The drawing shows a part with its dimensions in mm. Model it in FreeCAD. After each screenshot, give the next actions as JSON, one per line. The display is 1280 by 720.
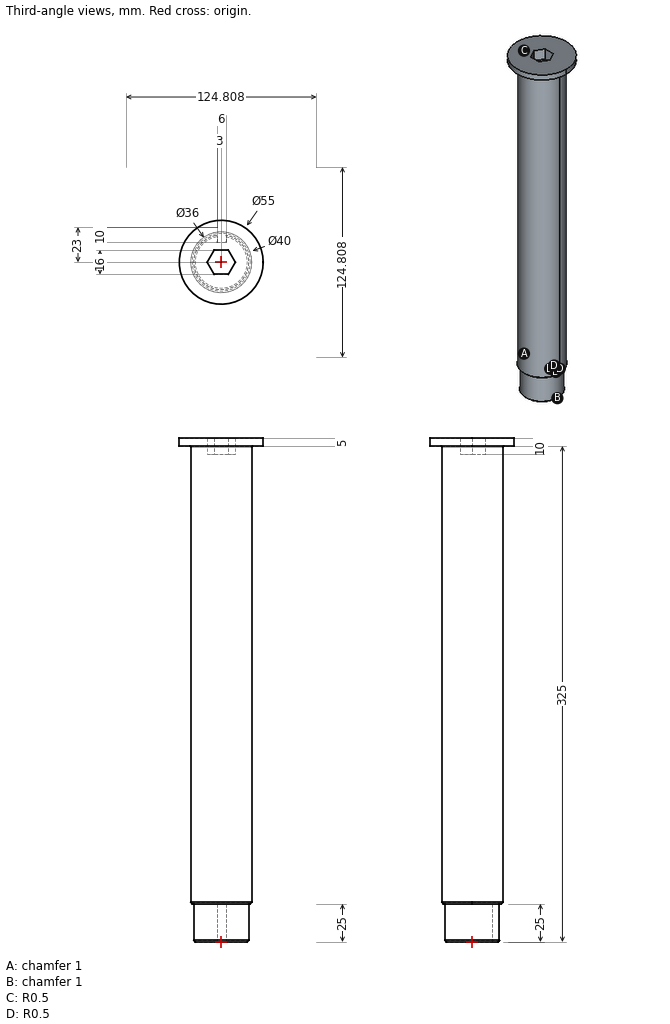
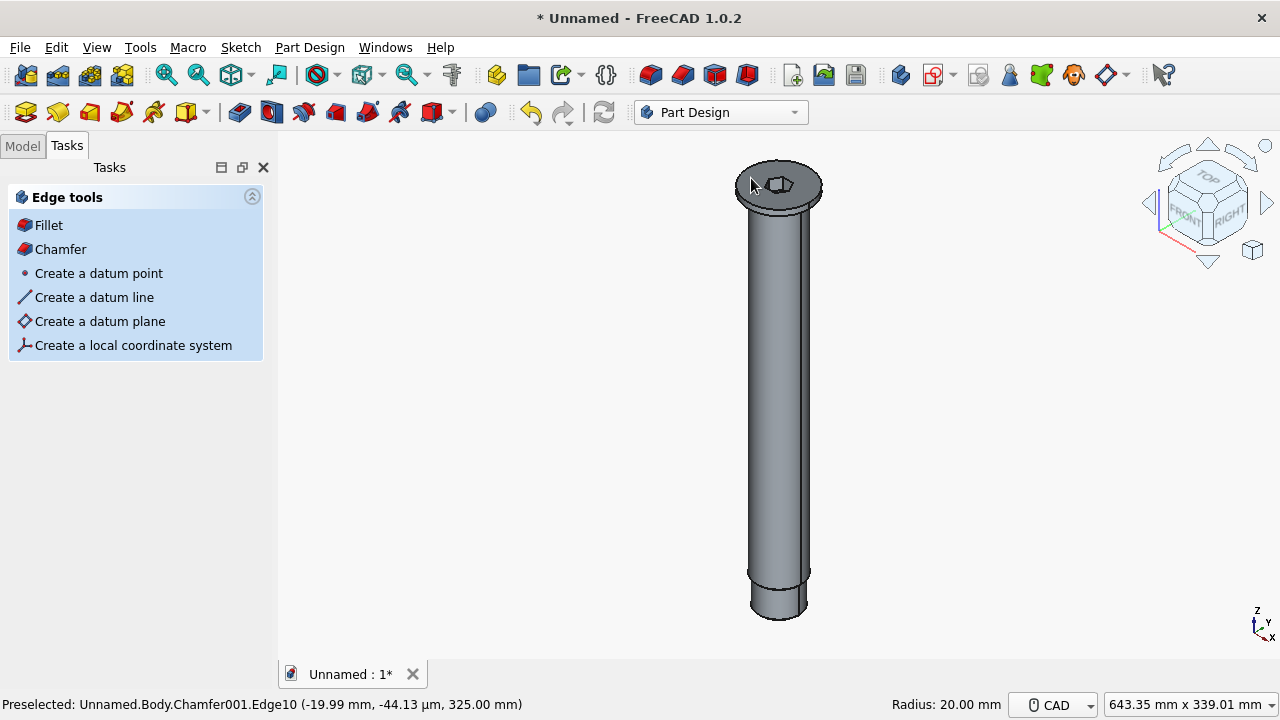
{"action": "left_click", "coordinate": [652, 76]}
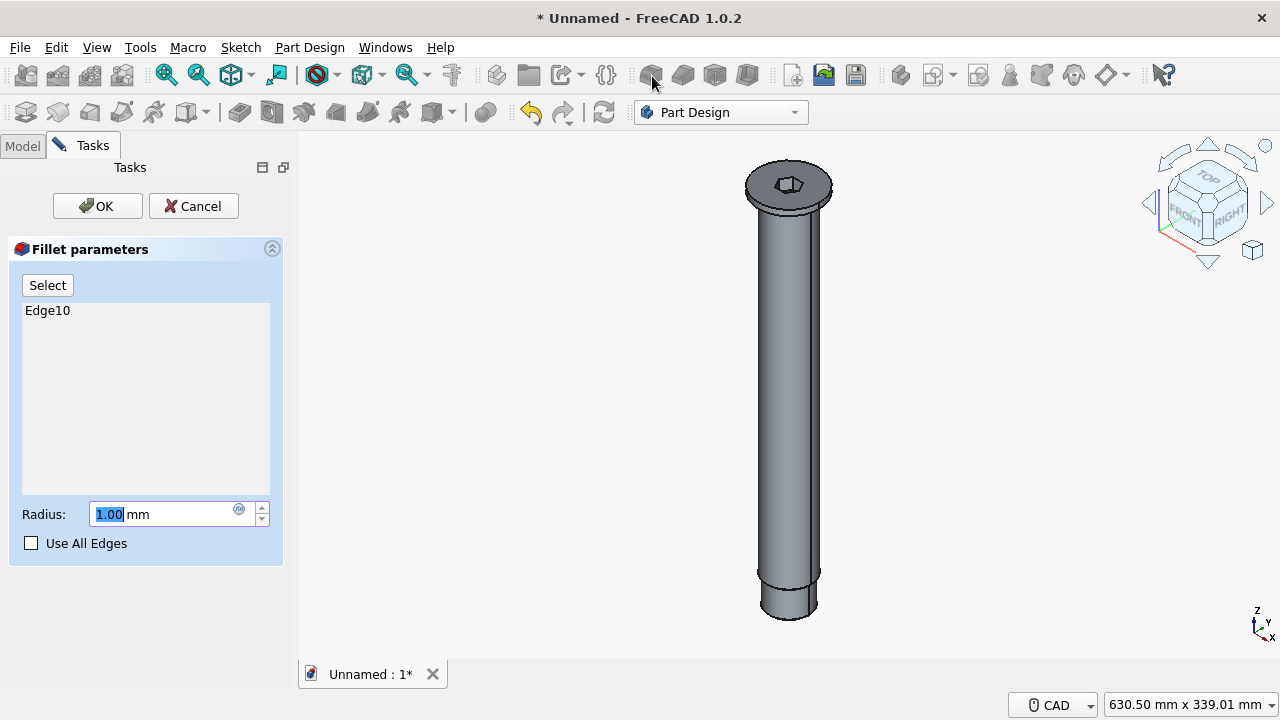
{"action": "type", "text": "0.5"}
{"action": "key", "text": "Tab"}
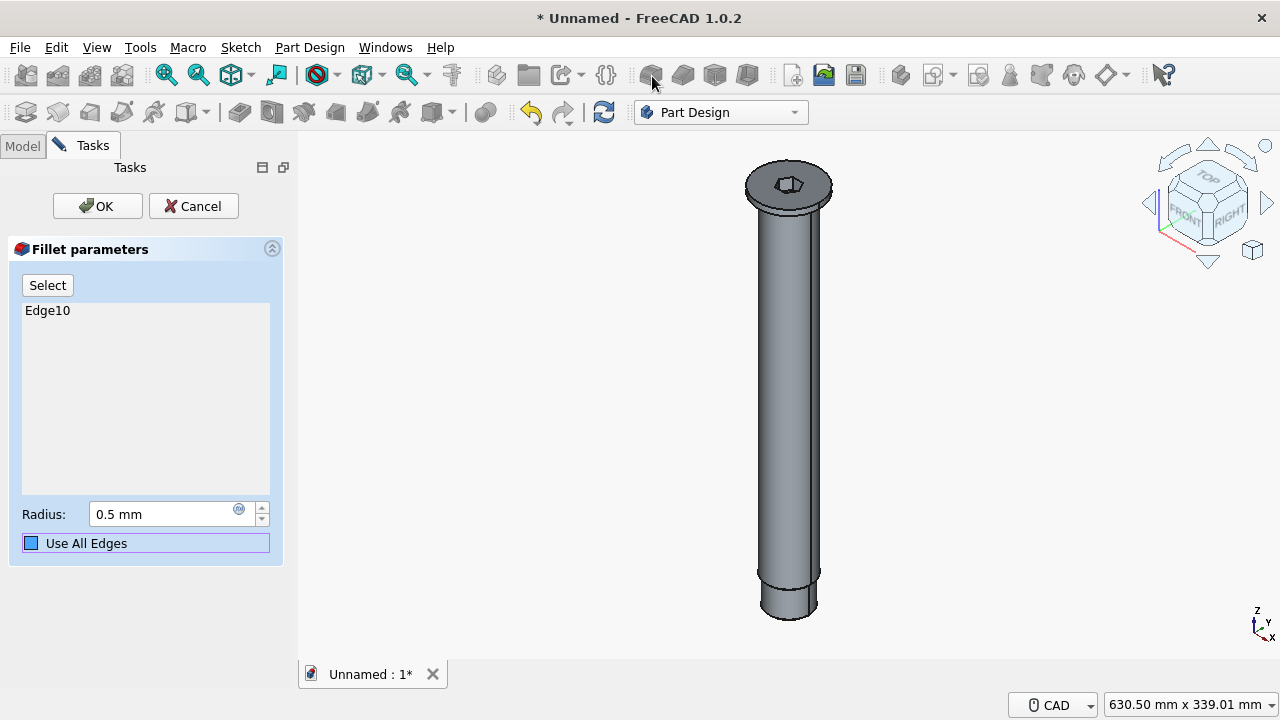
{"action": "left_click", "coordinate": [98, 206]}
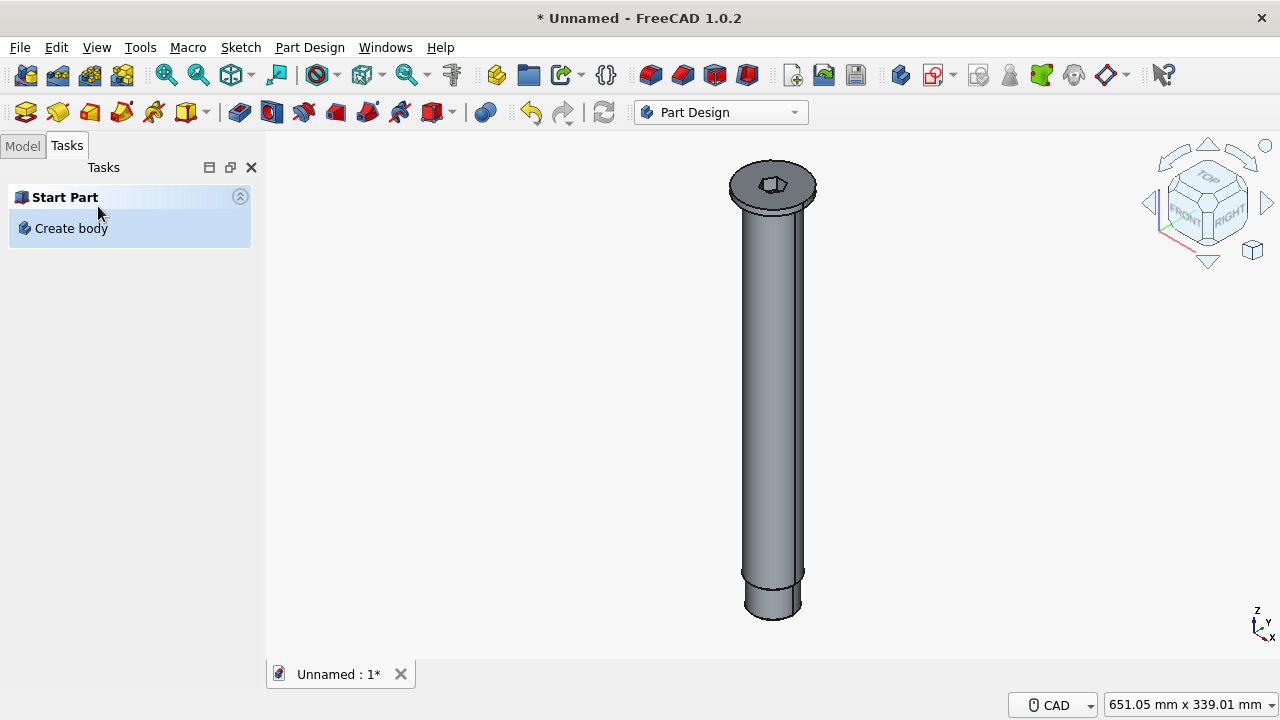
{"action": "left_click", "coordinate": [934, 76]}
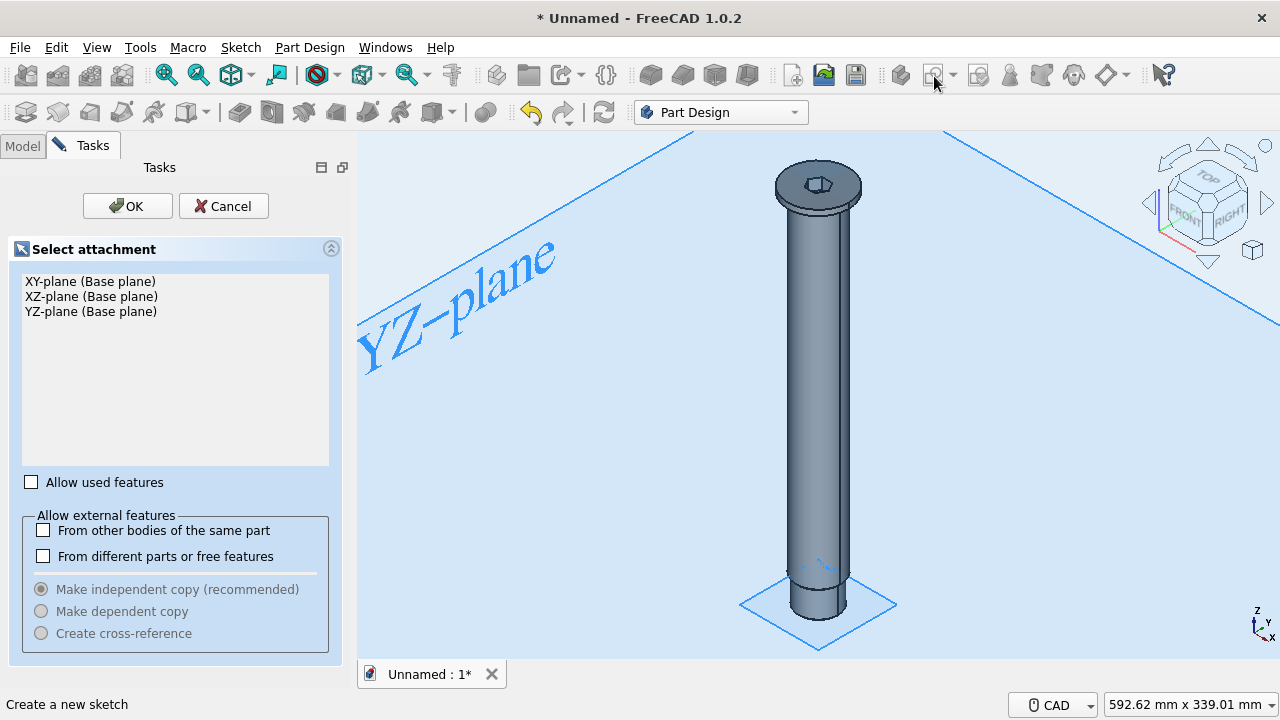
{"action": "left_click", "coordinate": [82, 282]}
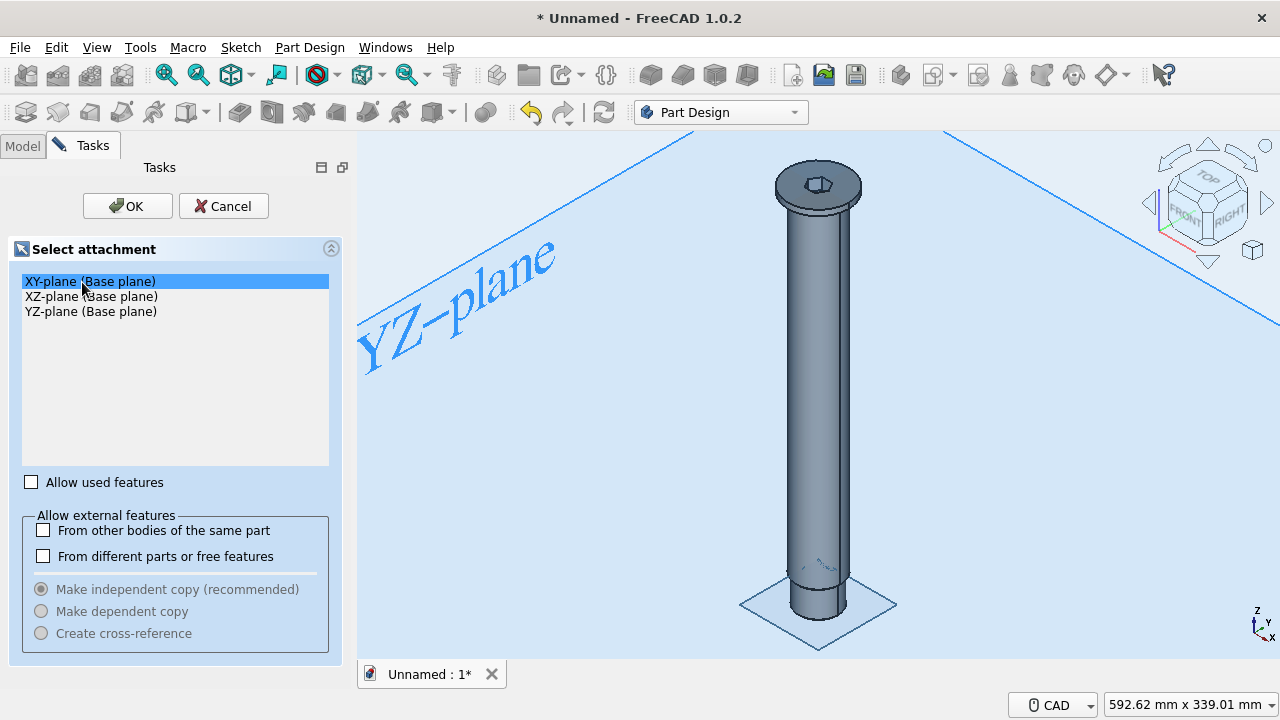
{"action": "left_click", "coordinate": [128, 206]}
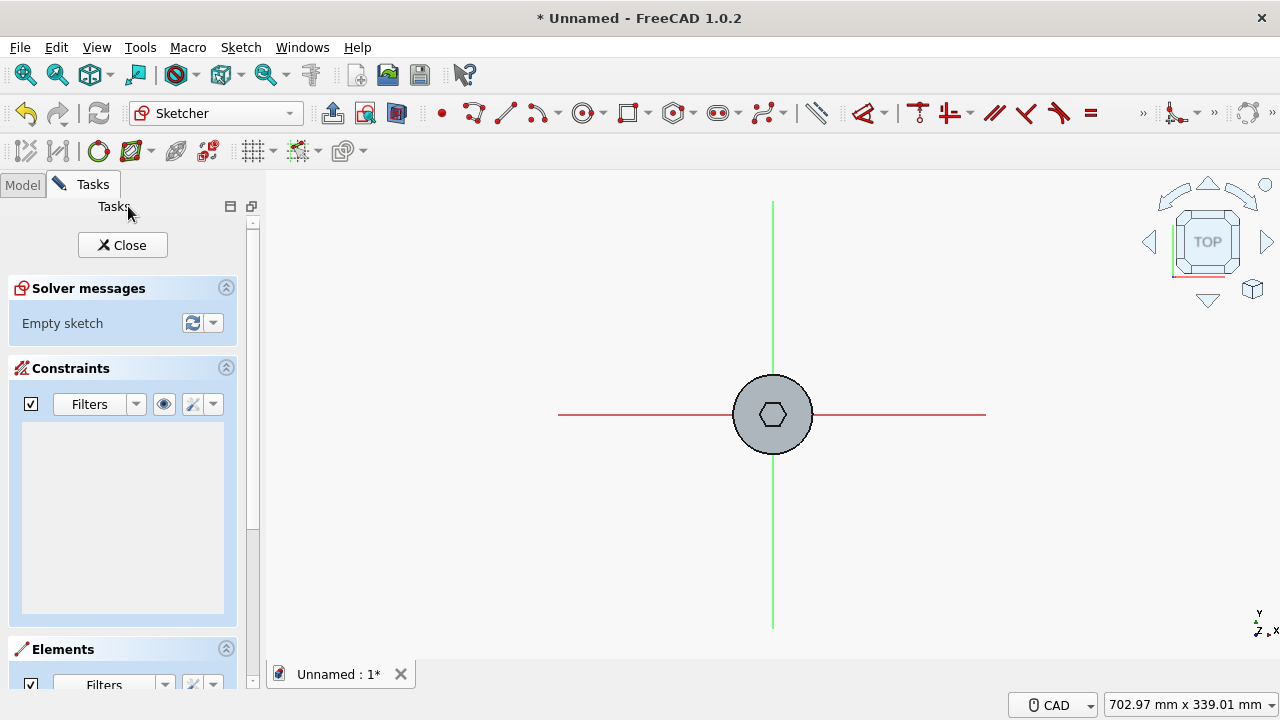
{"action": "left_click", "coordinate": [398, 114]}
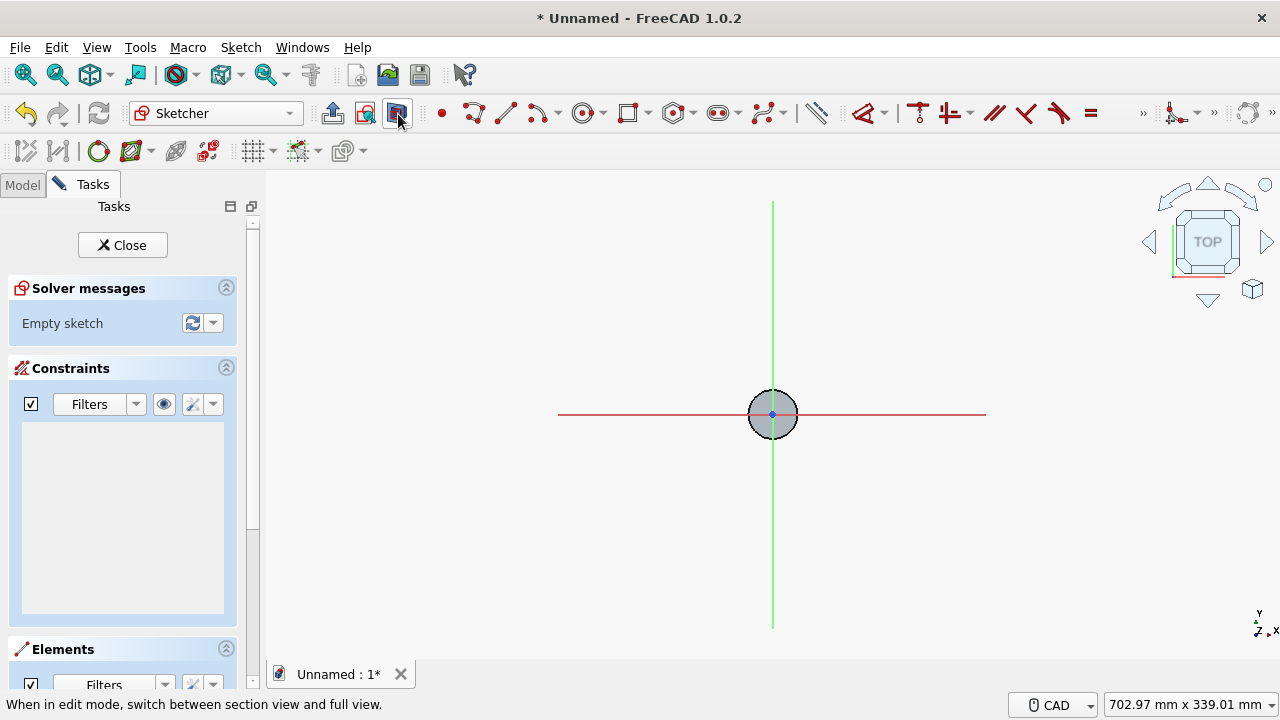
{"action": "scroll", "coordinate": [781, 396], "scroll_direction": "up", "scroll_amount": 11}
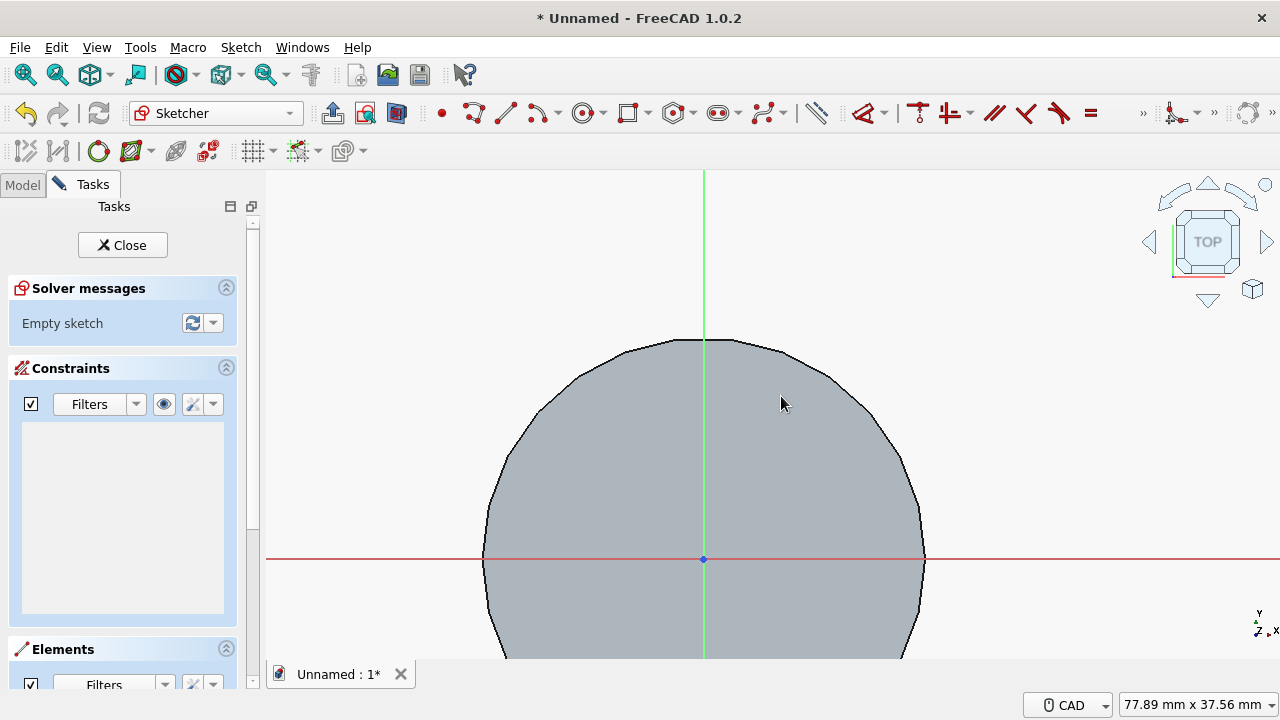
{"action": "left_click", "coordinate": [628, 114]}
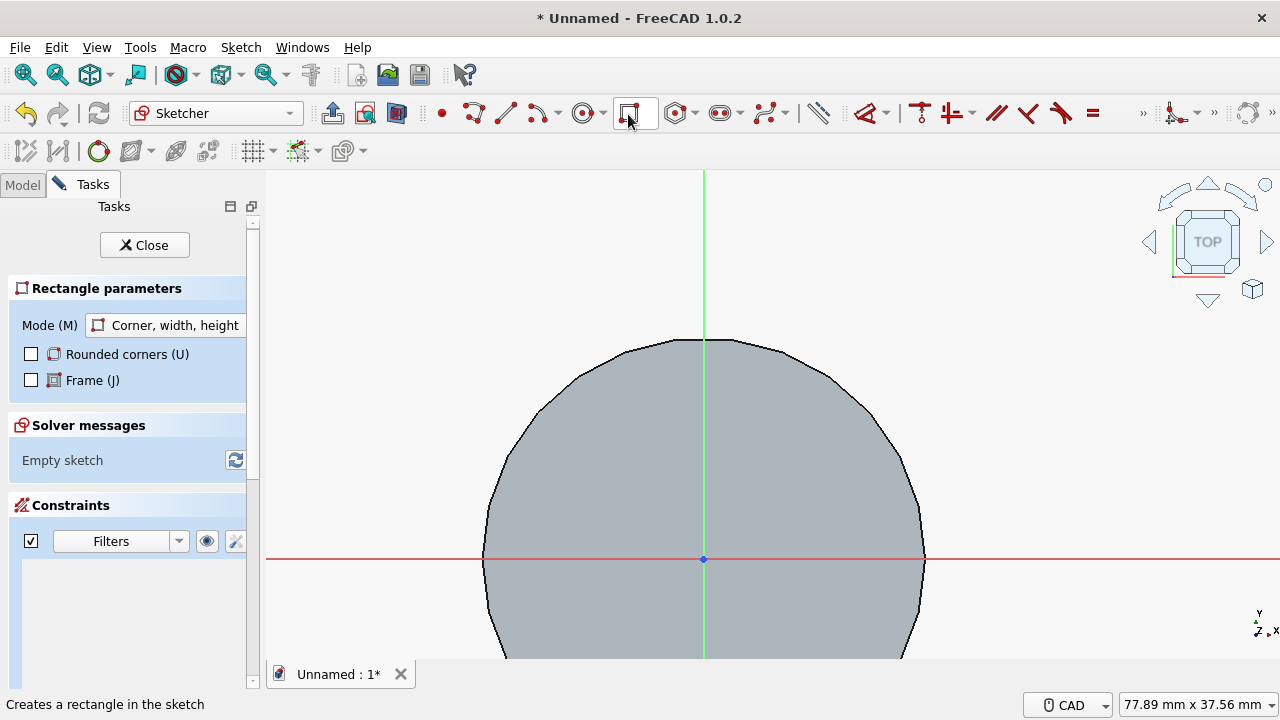
{"action": "left_click", "coordinate": [665, 260]}
{"action": "left_click", "coordinate": [743, 390]}
{"action": "key", "text": "Escape"}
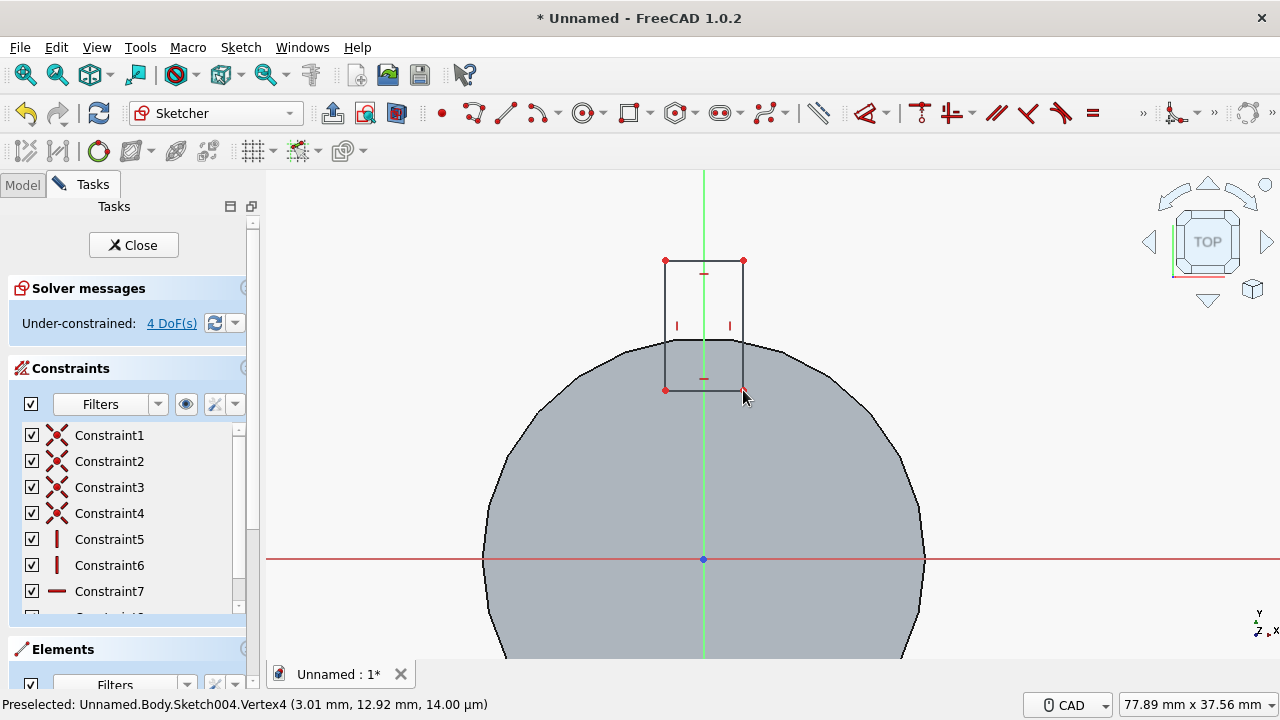
{"action": "left_click", "coordinate": [866, 114]}